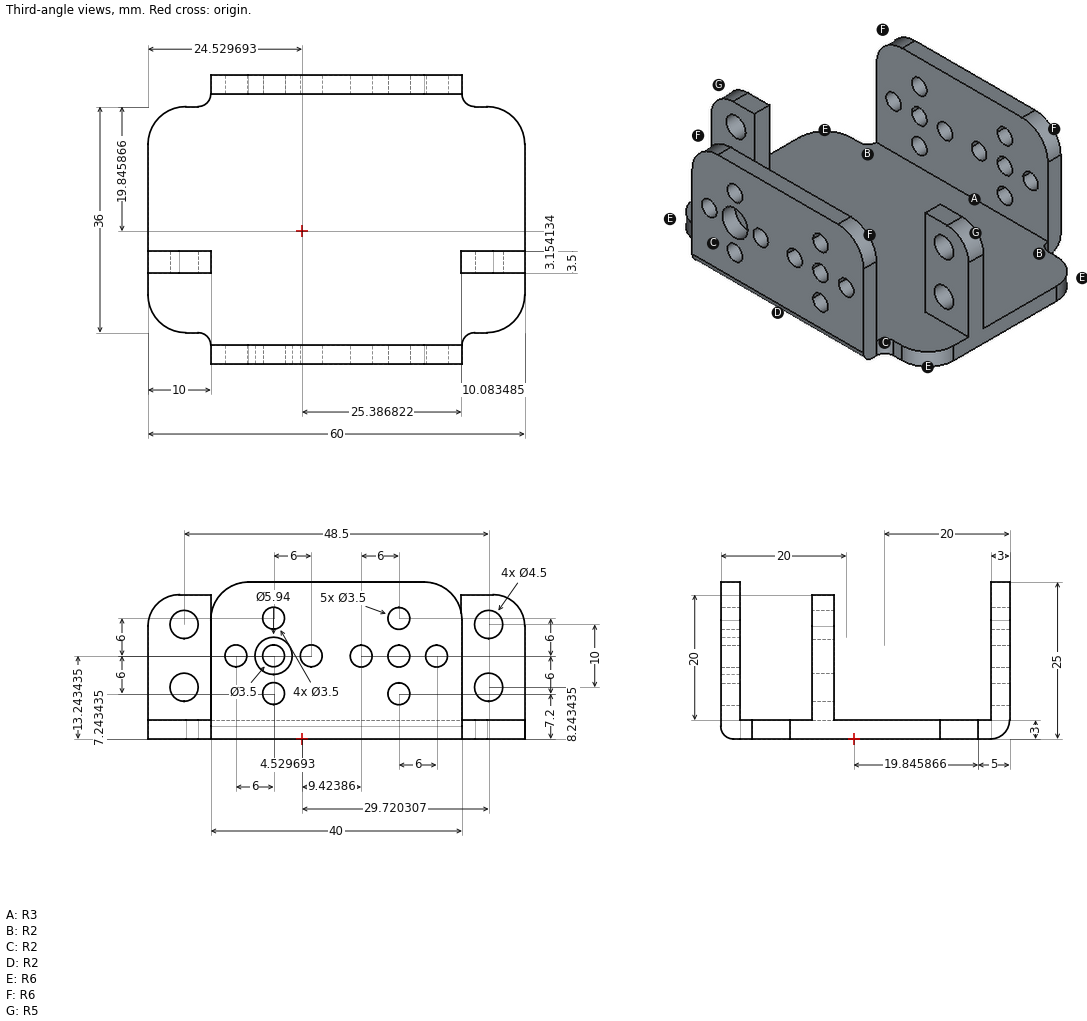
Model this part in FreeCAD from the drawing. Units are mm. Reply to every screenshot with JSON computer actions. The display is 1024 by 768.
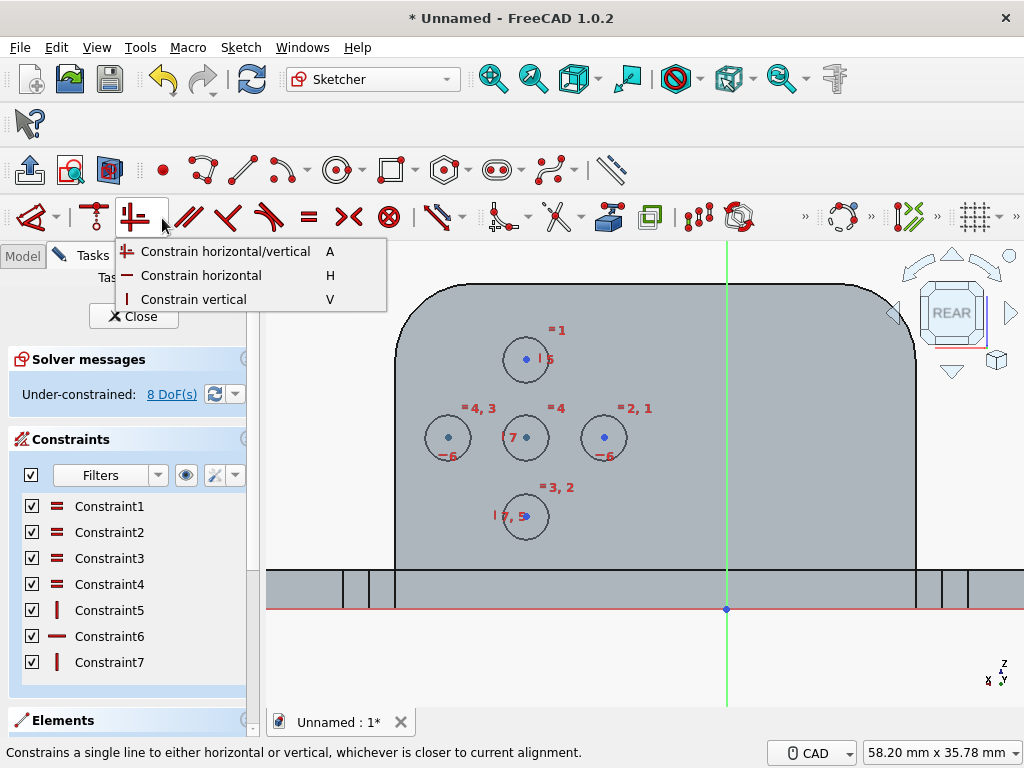
{"action": "left_click", "coordinate": [251, 275]}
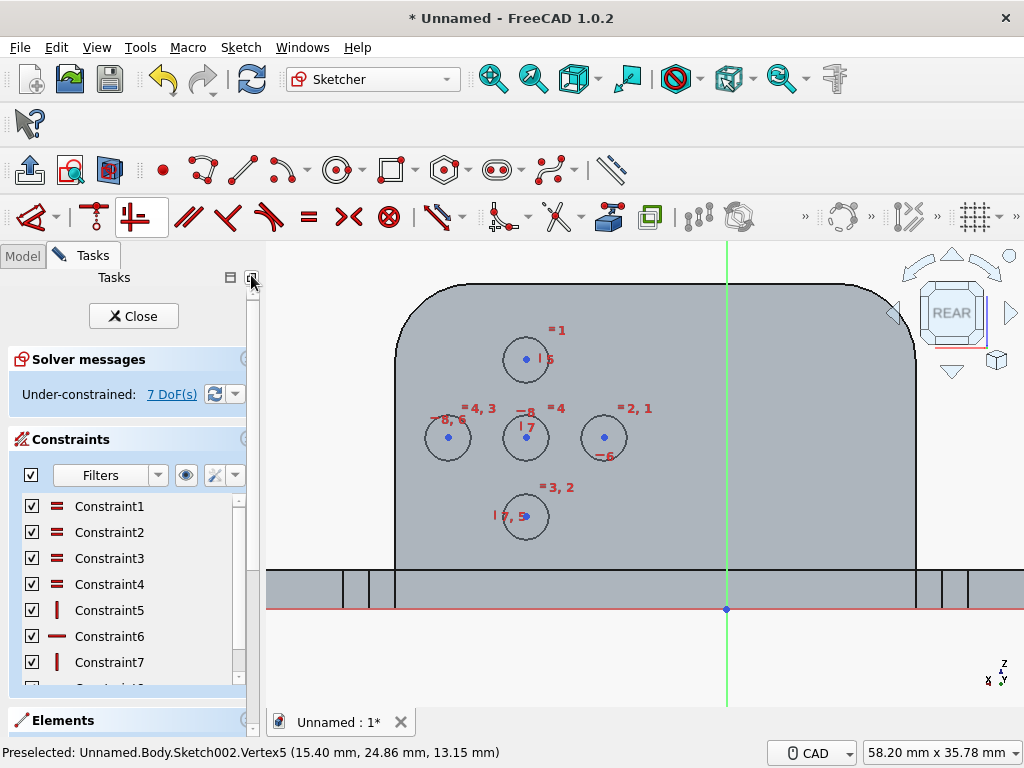
{"action": "left_click", "coordinate": [32, 218]}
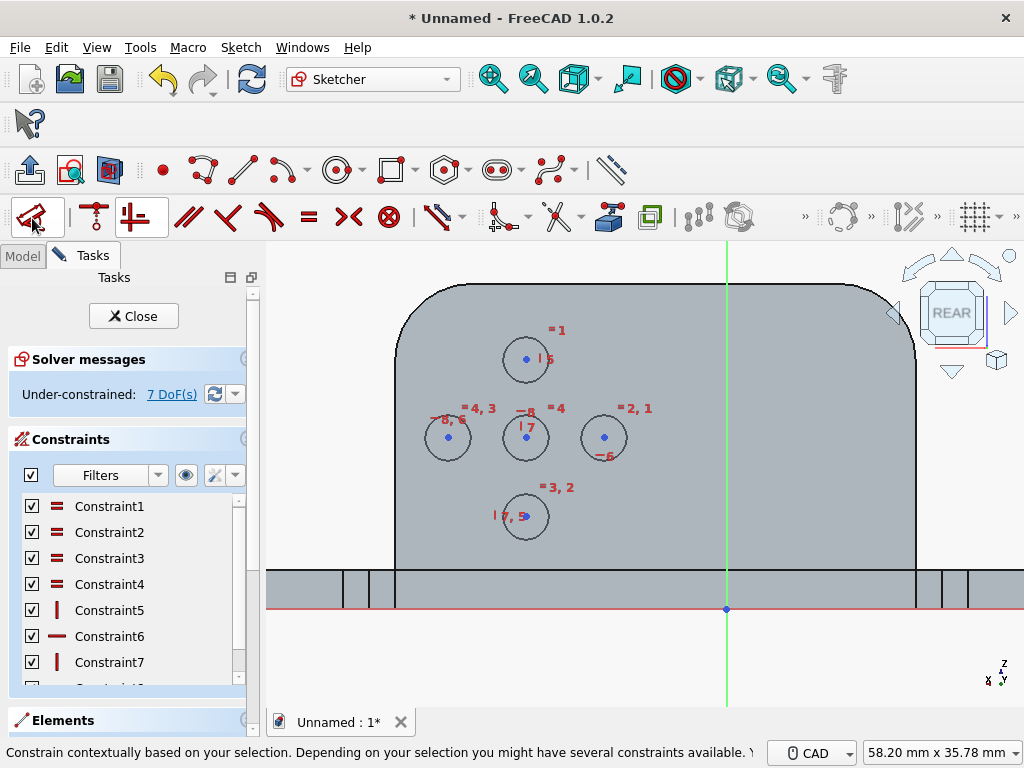
{"action": "left_click", "coordinate": [542, 344]}
{"action": "left_click", "coordinate": [565, 321]}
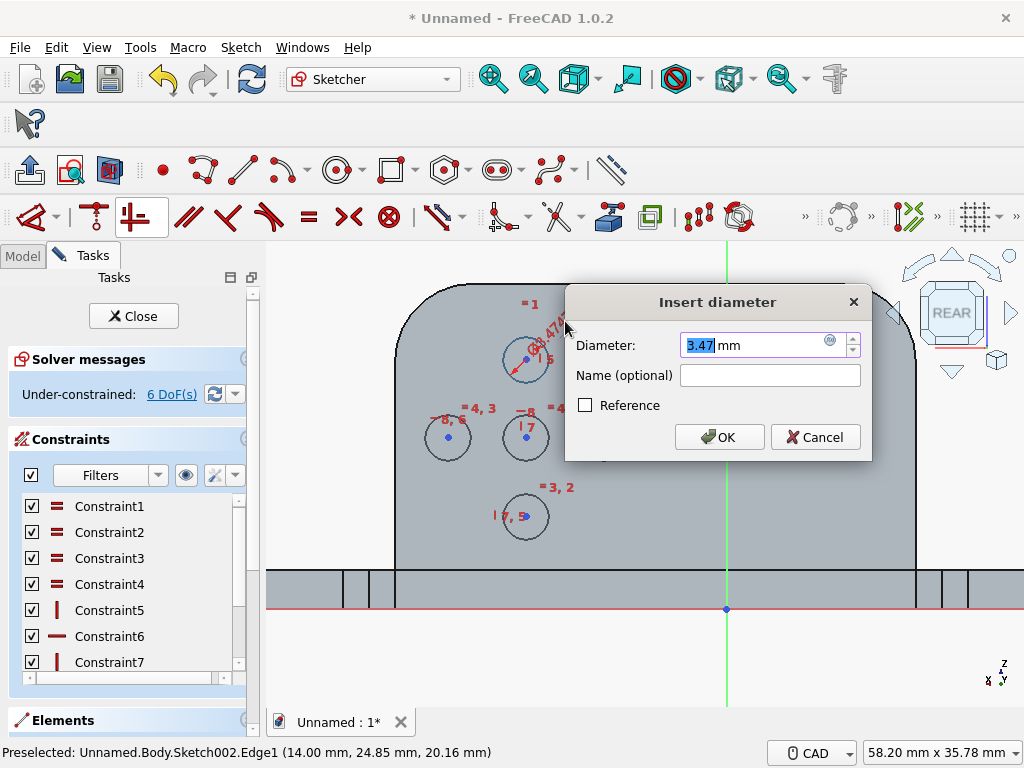
{"action": "type", "text": "3.5"}
{"action": "key", "text": "Return"}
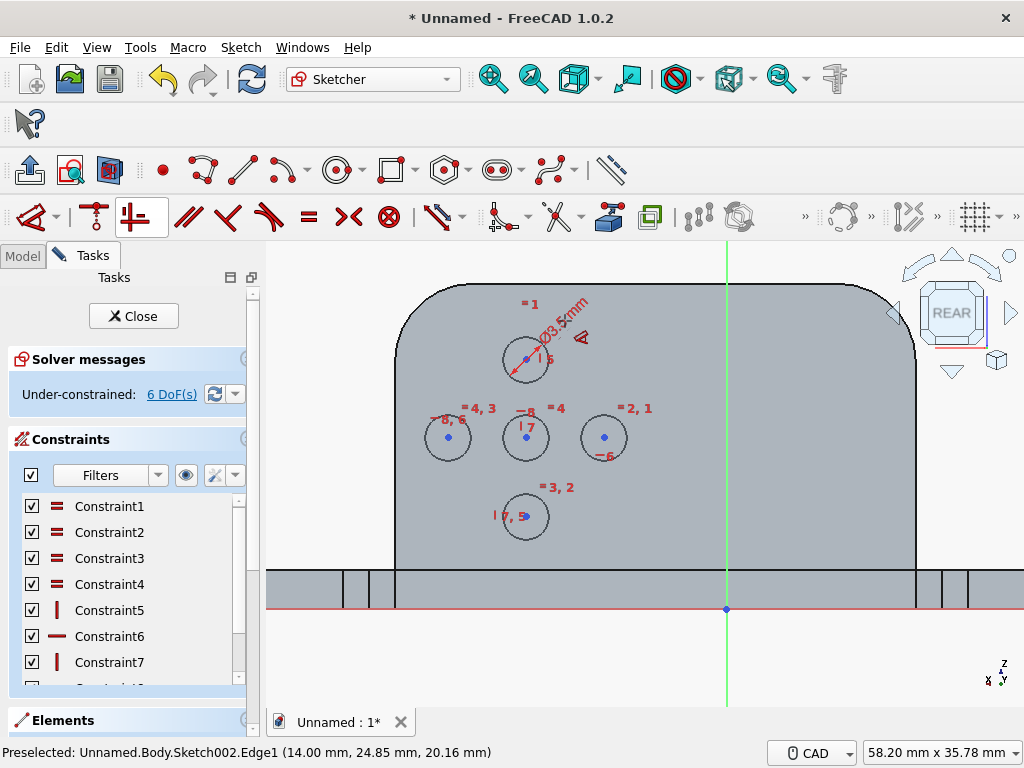
{"action": "left_click", "coordinate": [526, 360]}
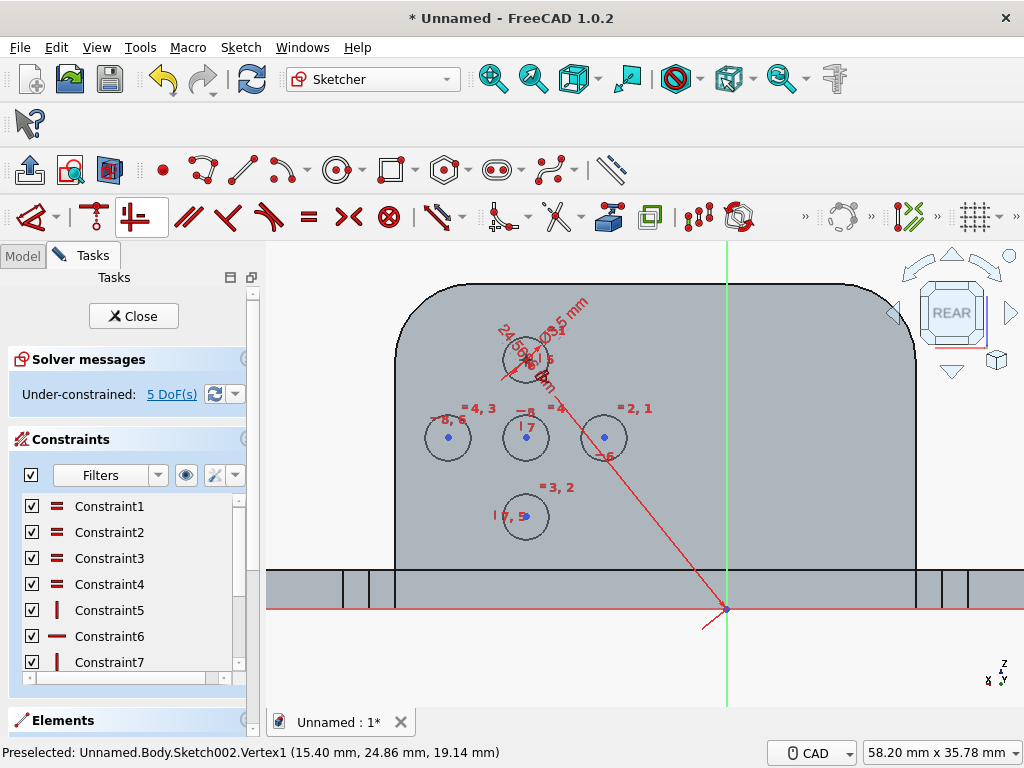
{"action": "left_click", "coordinate": [604, 438]}
{"action": "left_click", "coordinate": [565, 472]}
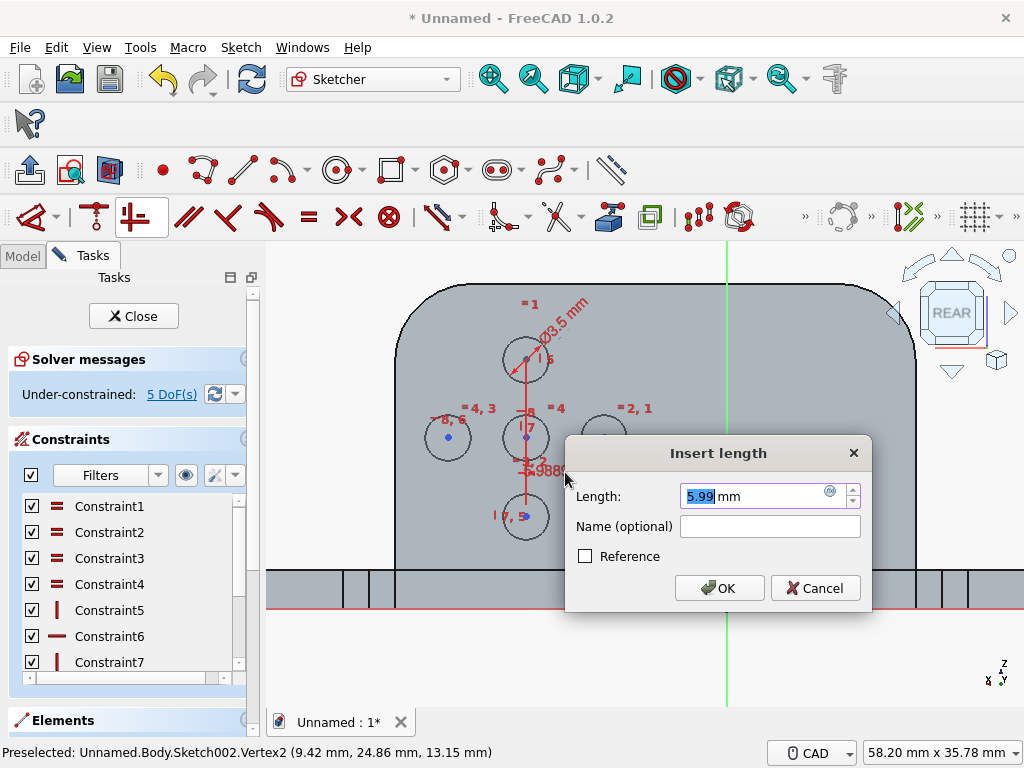
{"action": "type", "text": "6"}
{"action": "key", "text": "Return"}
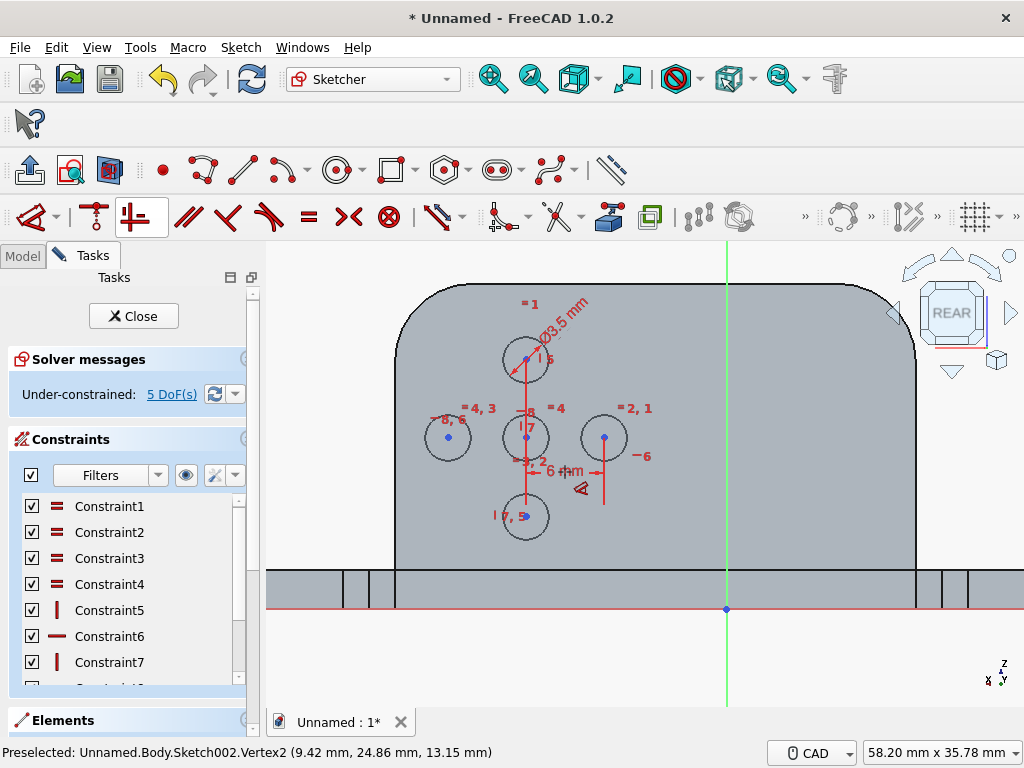
{"action": "left_click", "coordinate": [526, 360]}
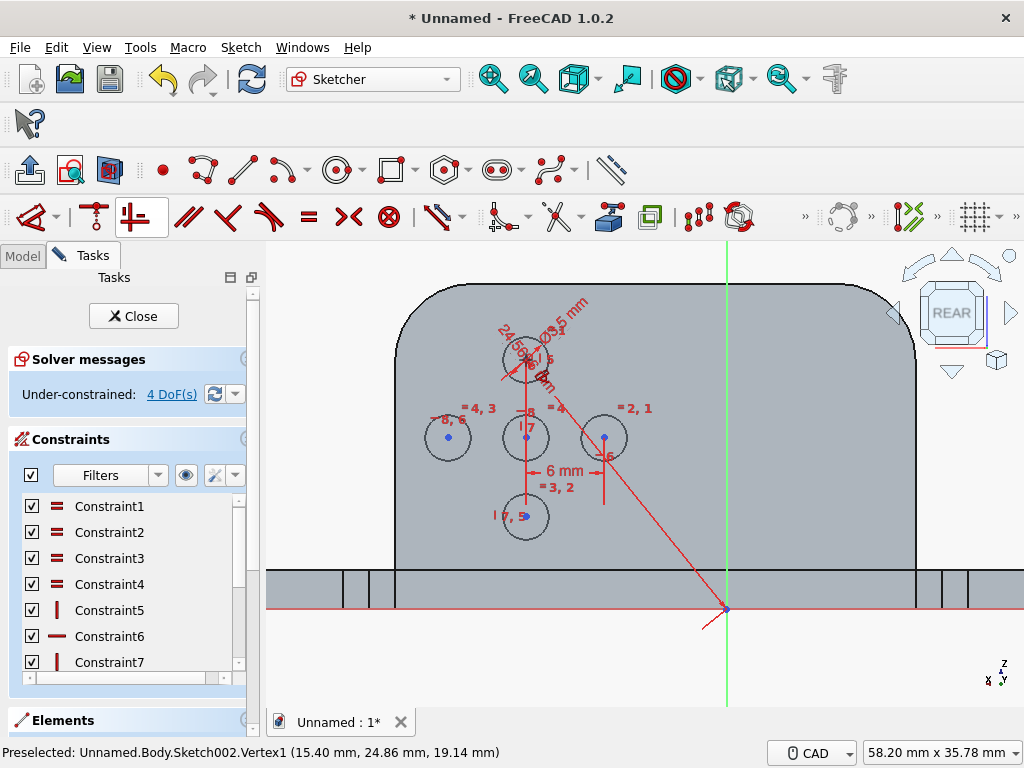
{"action": "left_click", "coordinate": [604, 438]}
{"action": "left_click", "coordinate": [492, 399]}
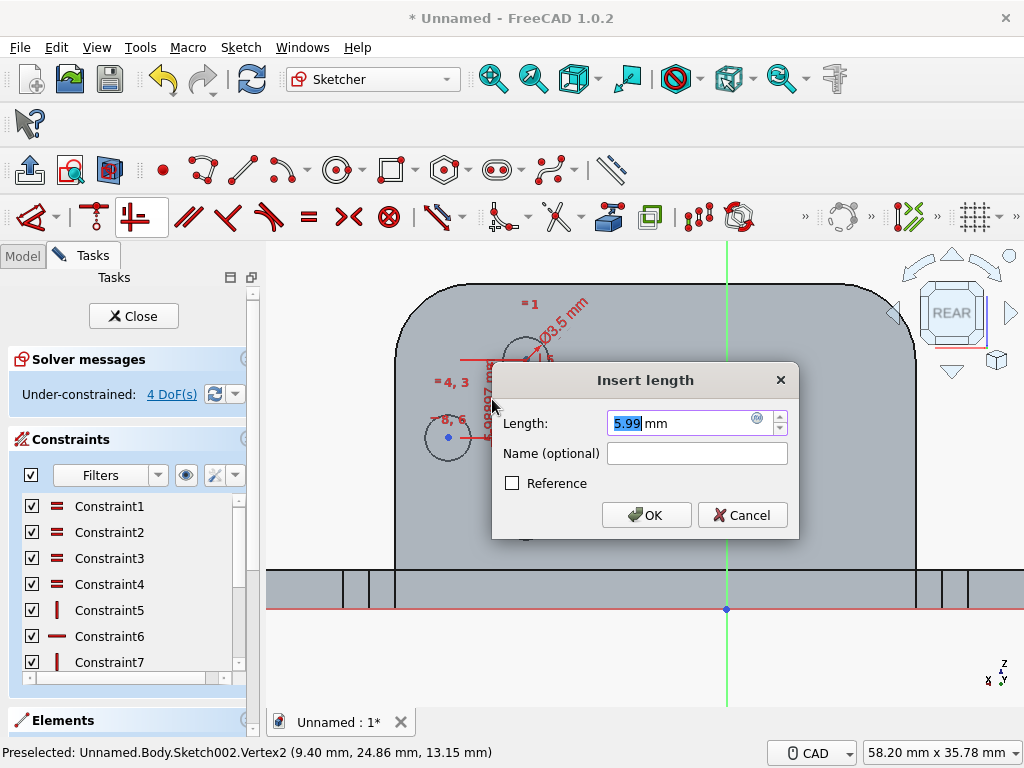
{"action": "type", "text": "6"}
{"action": "key", "text": "Return"}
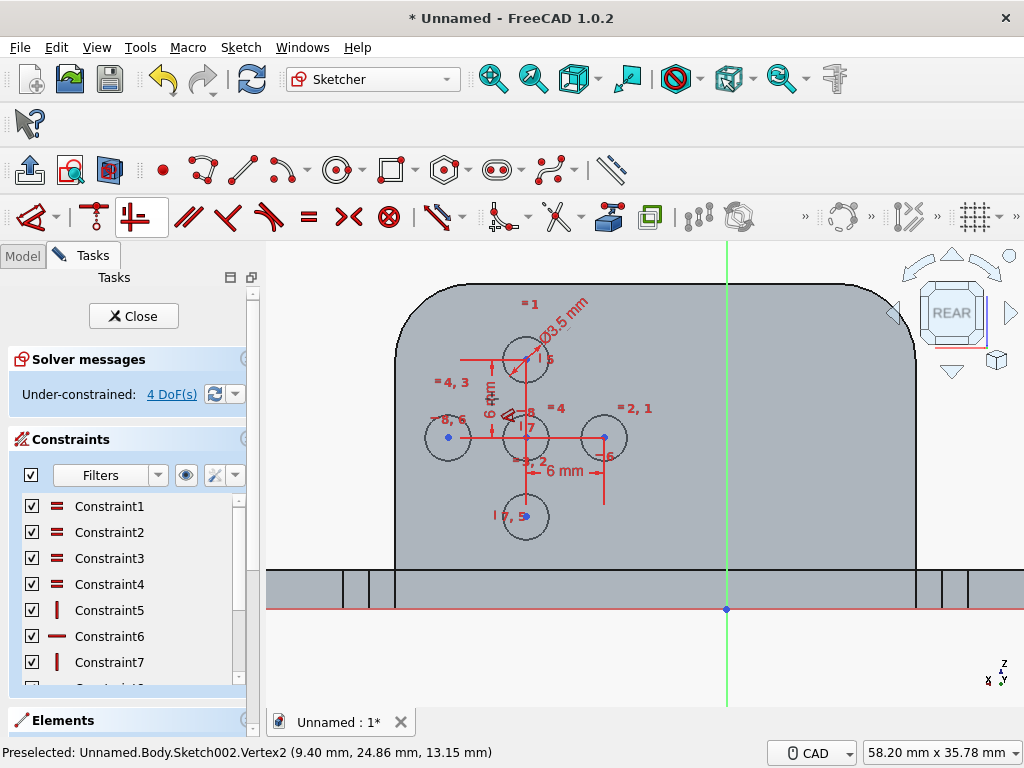
{"action": "left_click", "coordinate": [604, 438]}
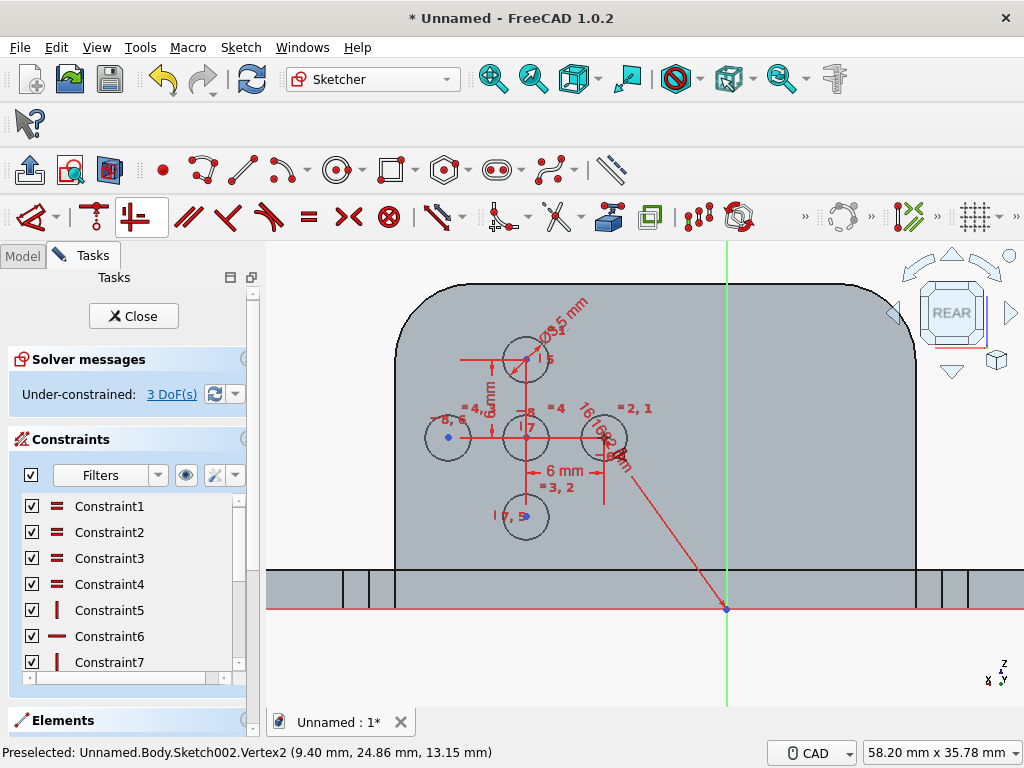
{"action": "left_click", "coordinate": [526, 517]}
{"action": "left_click", "coordinate": [492, 477]}